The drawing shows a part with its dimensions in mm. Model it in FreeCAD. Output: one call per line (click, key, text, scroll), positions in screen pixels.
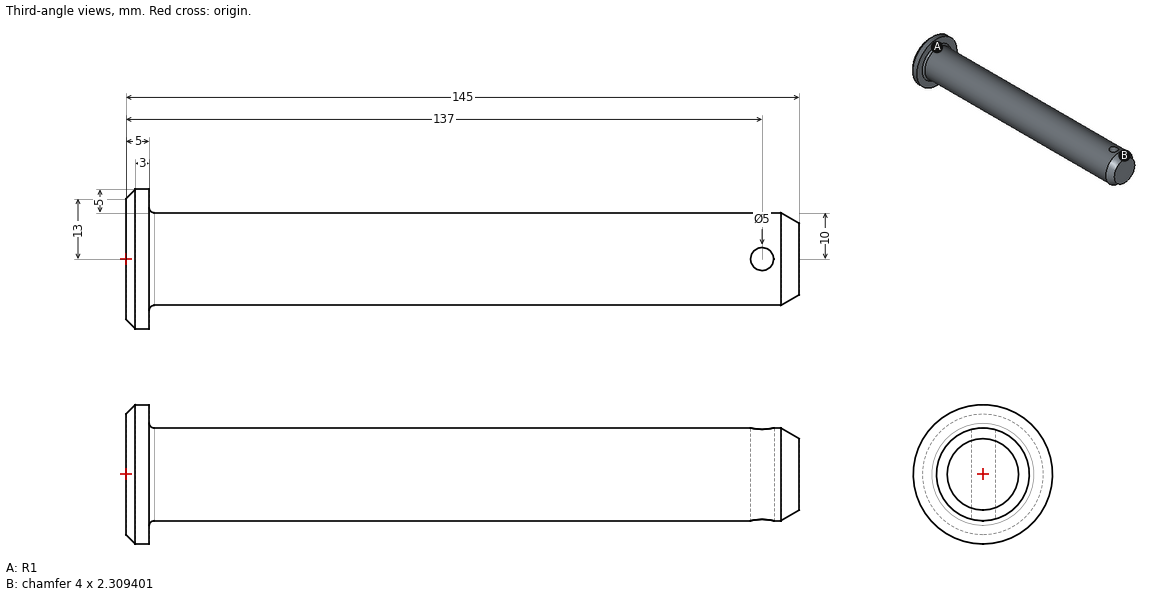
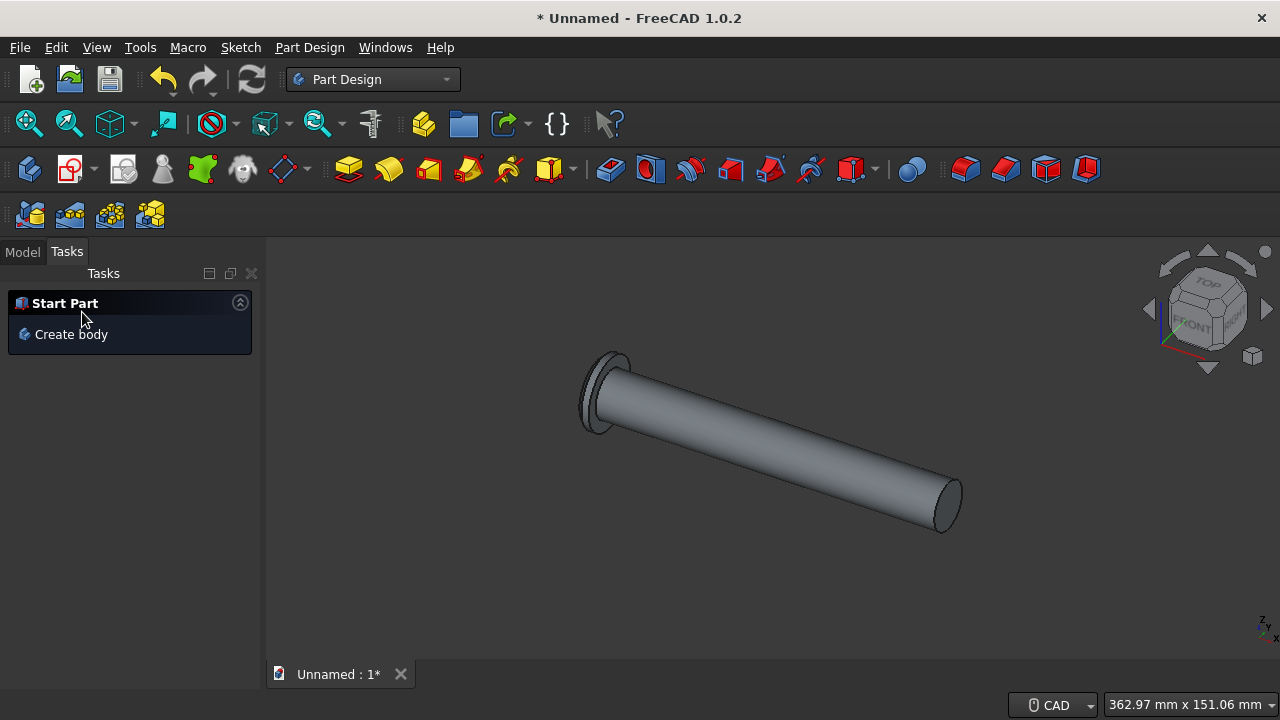
click(70, 170)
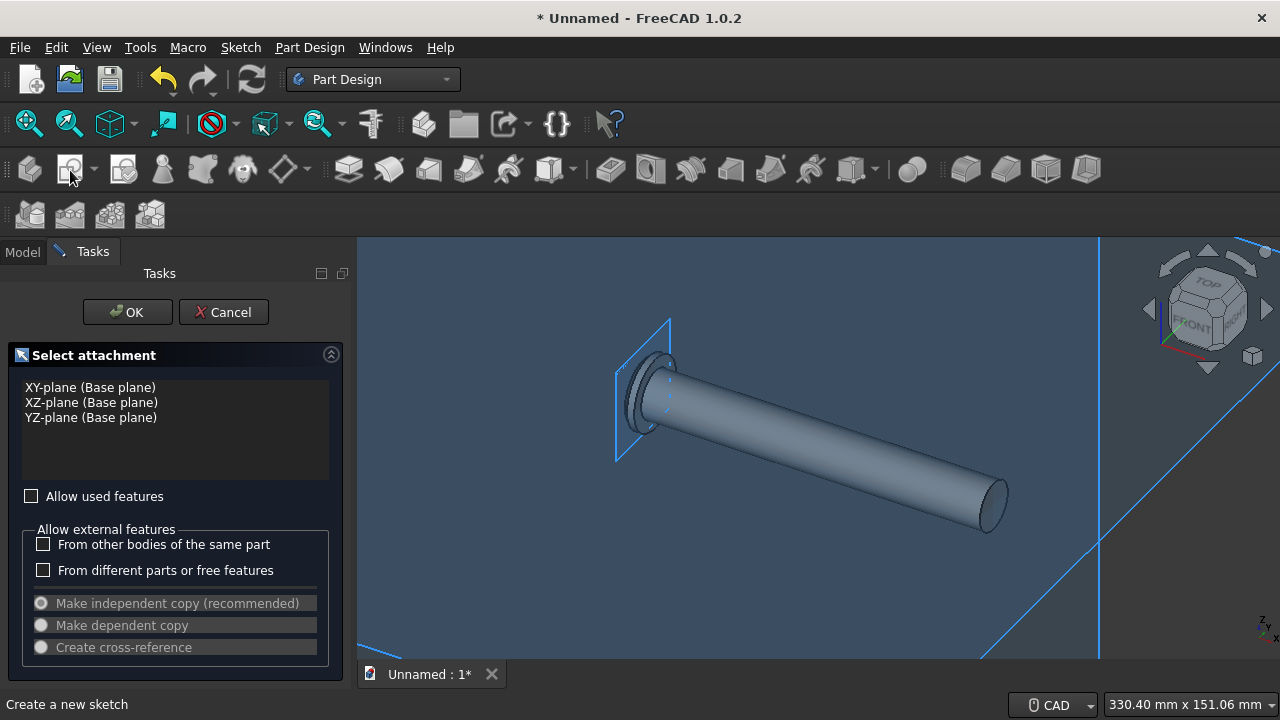
click(82, 388)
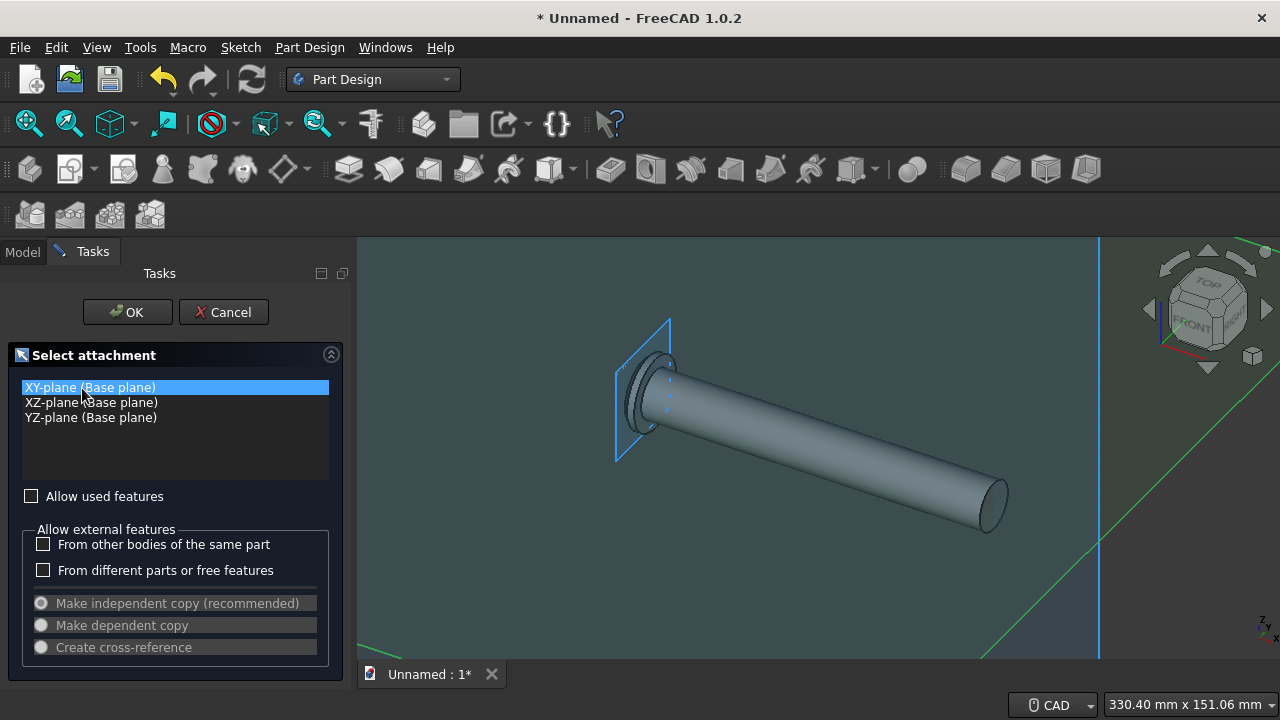
click(128, 312)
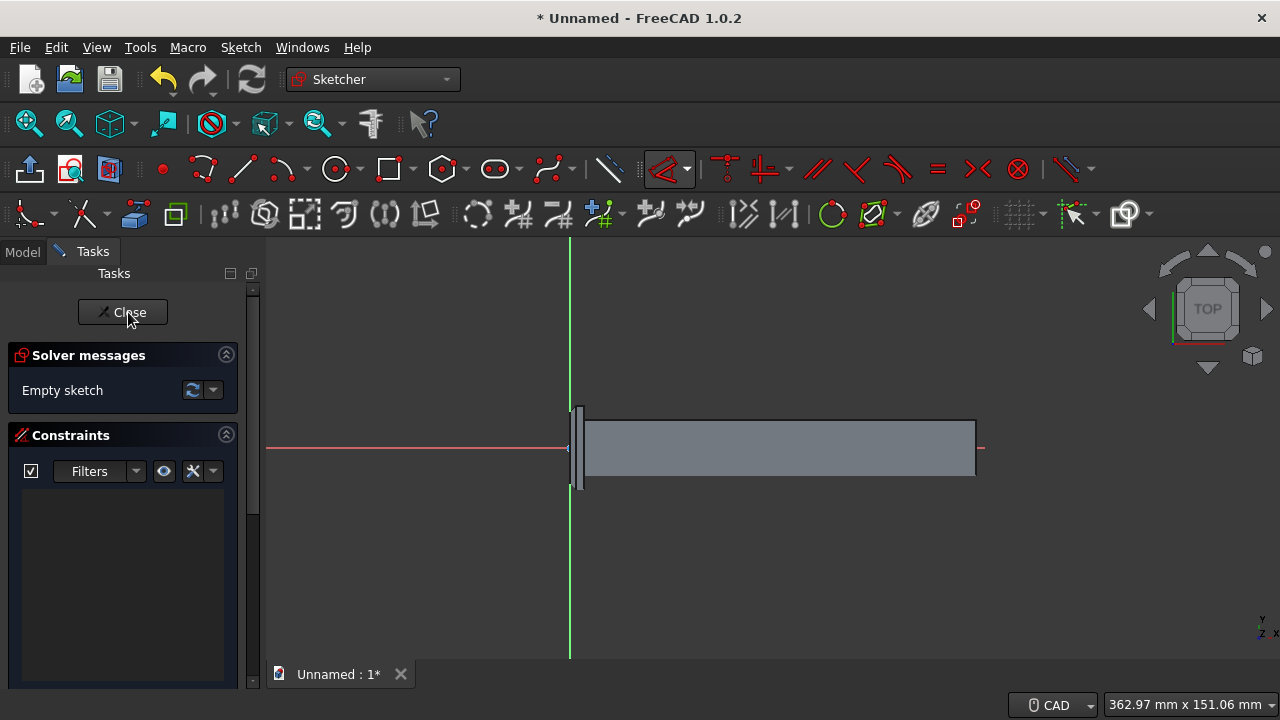
click(110, 170)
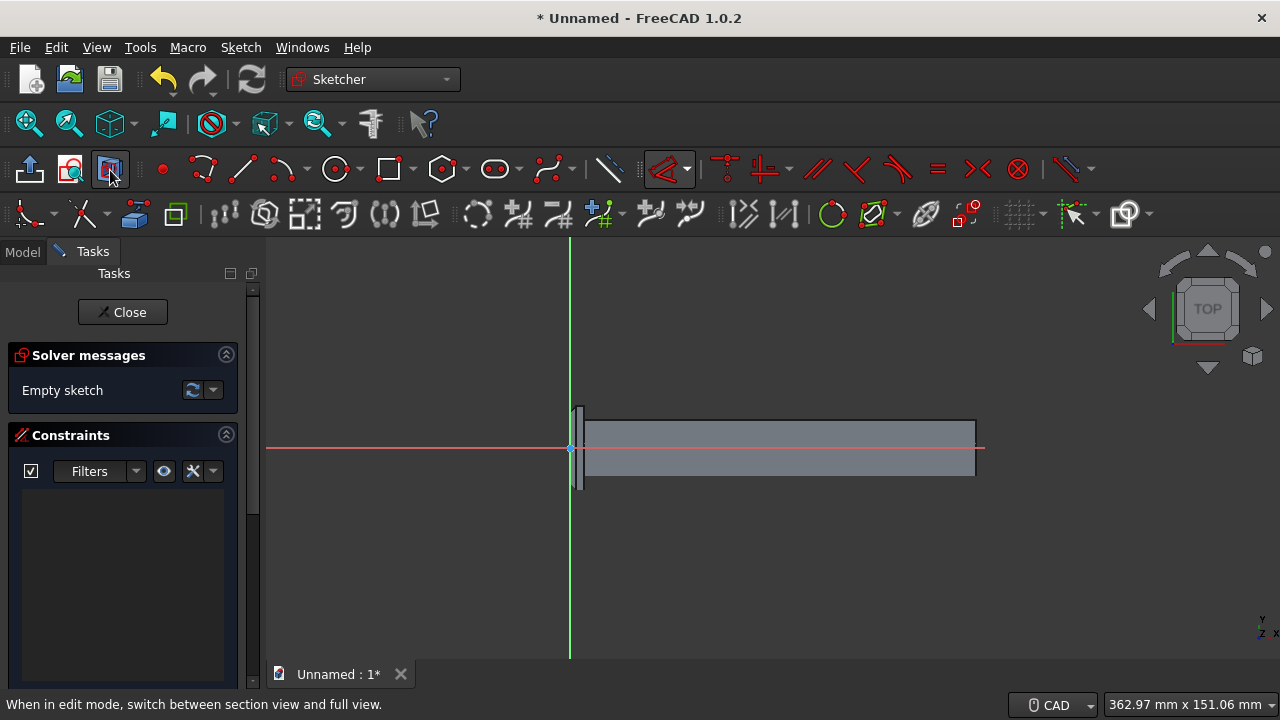
scroll(966, 448, up, 15)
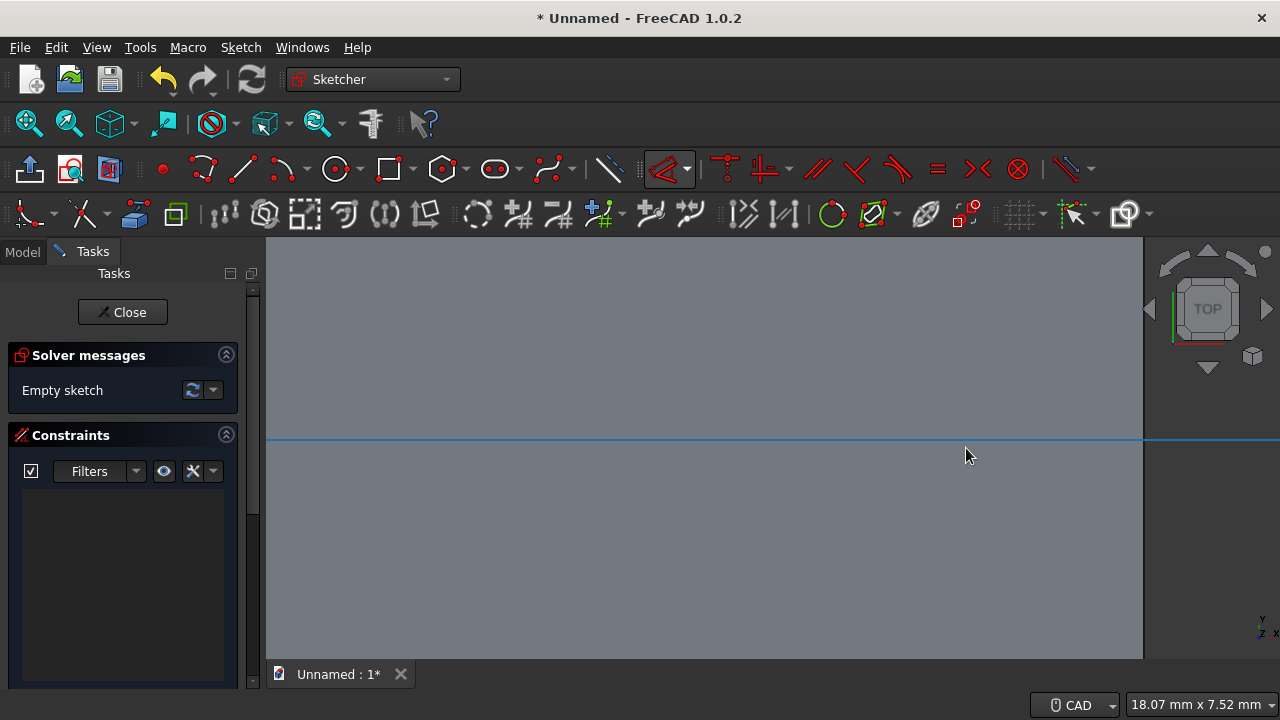
key(g)
key(c)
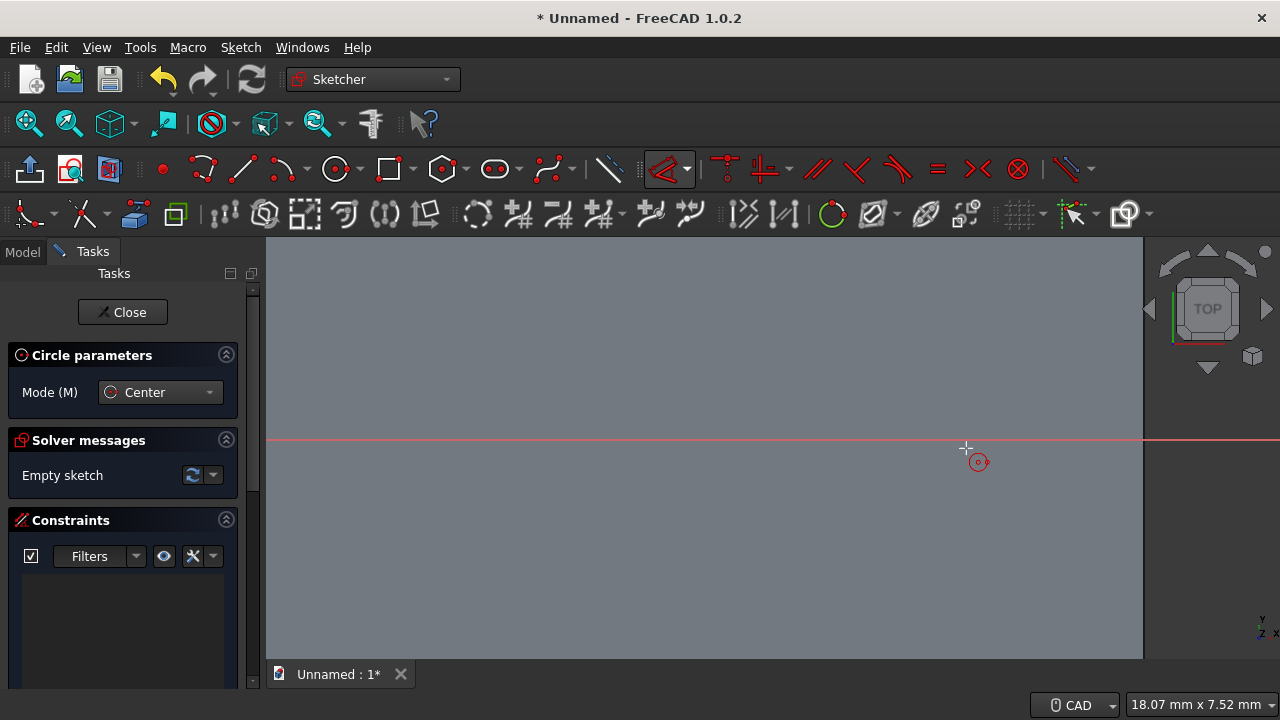
click(695, 440)
click(795, 341)
key(Escape)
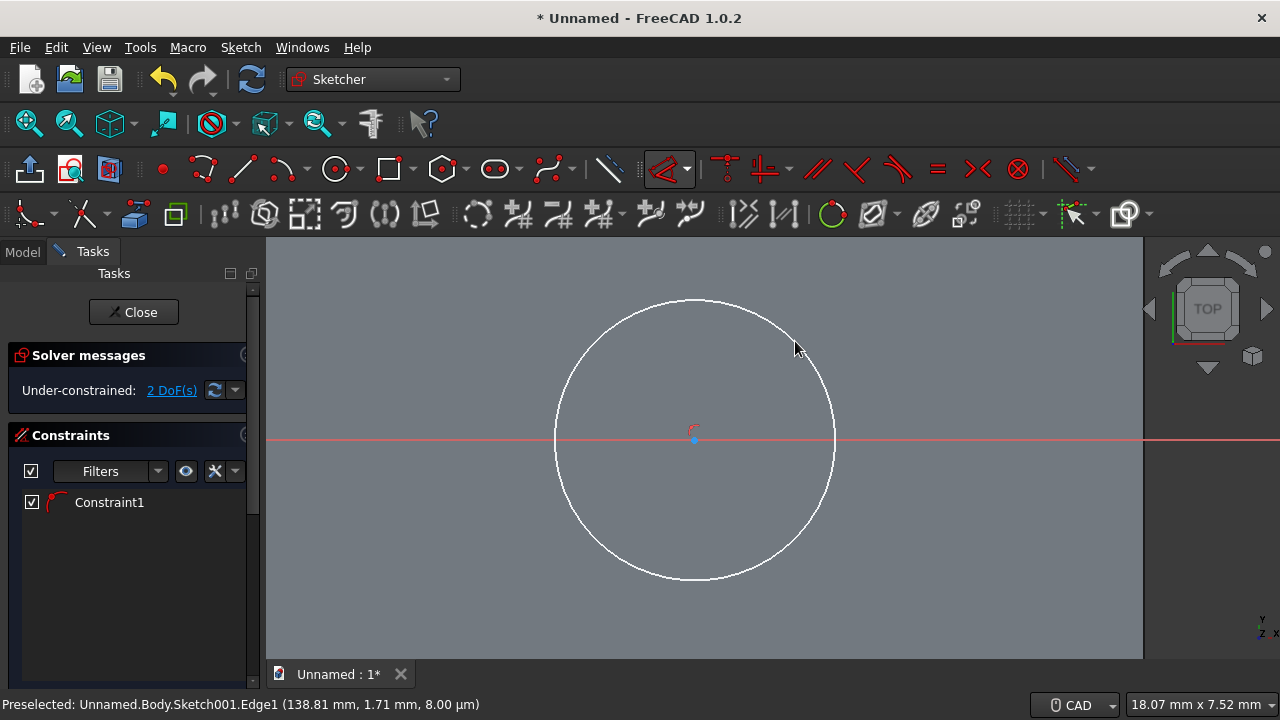
click(794, 341)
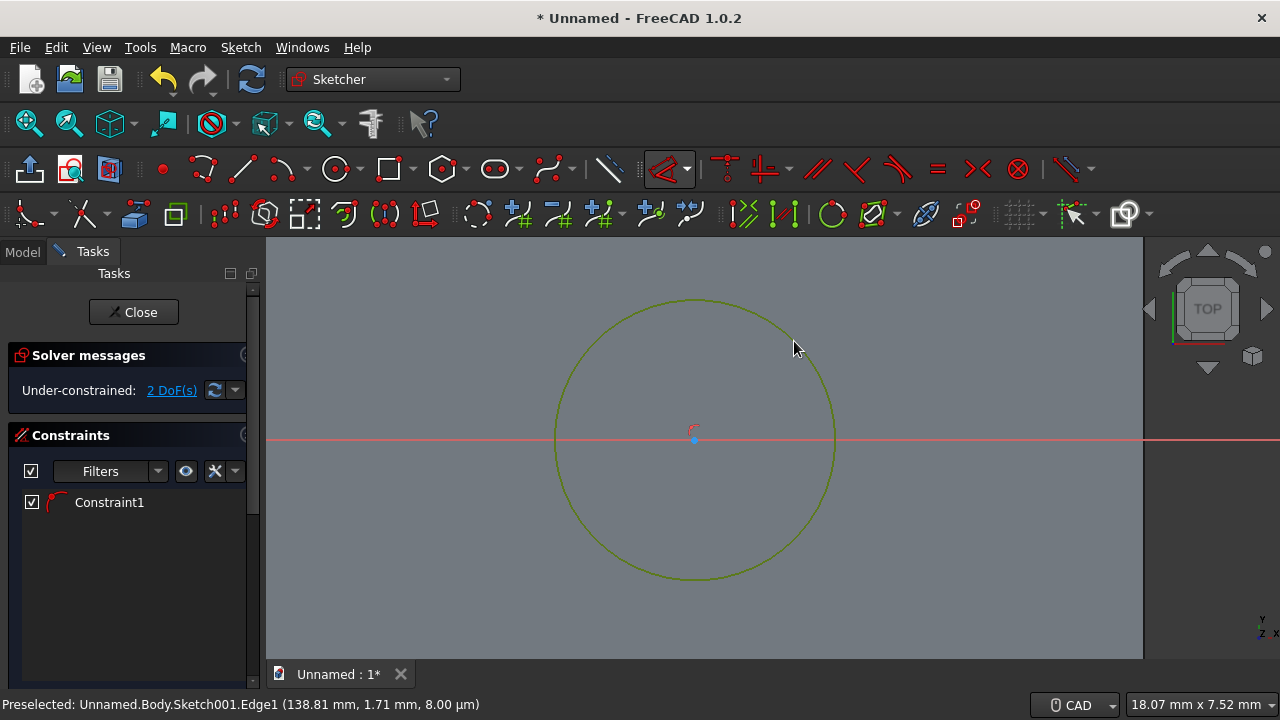
key(k)
key(o)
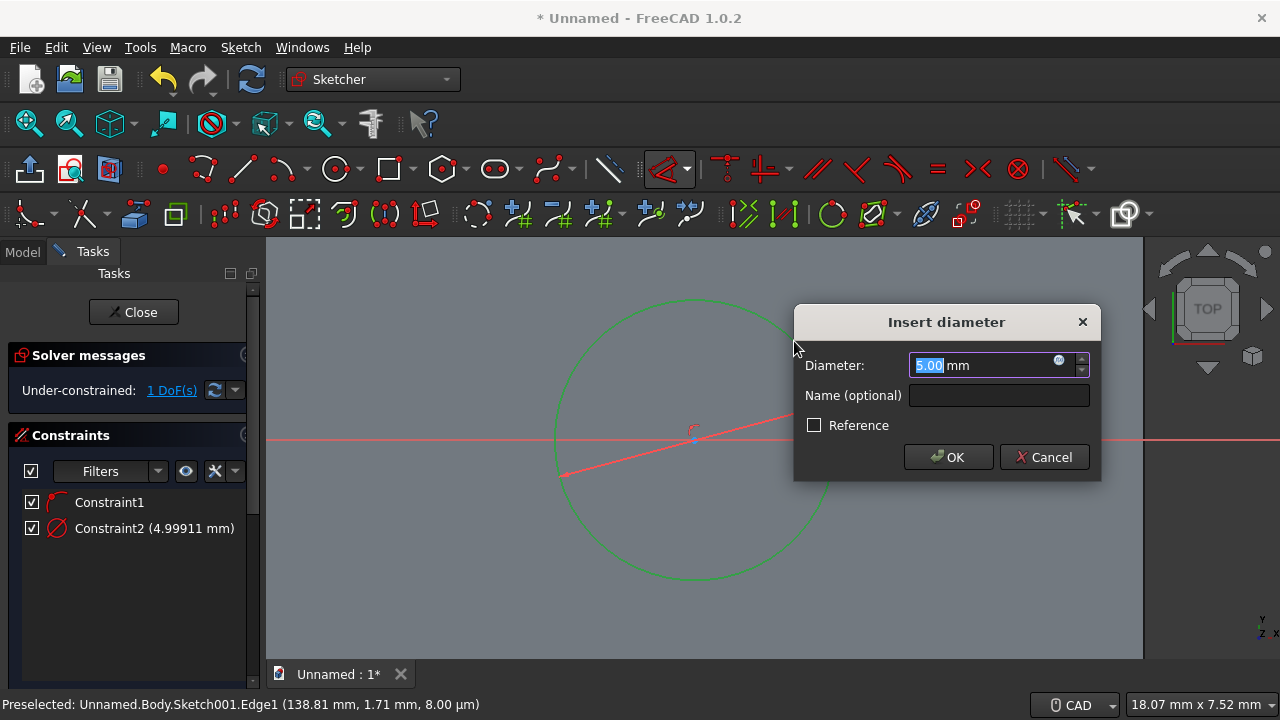
text(5)
key(Return)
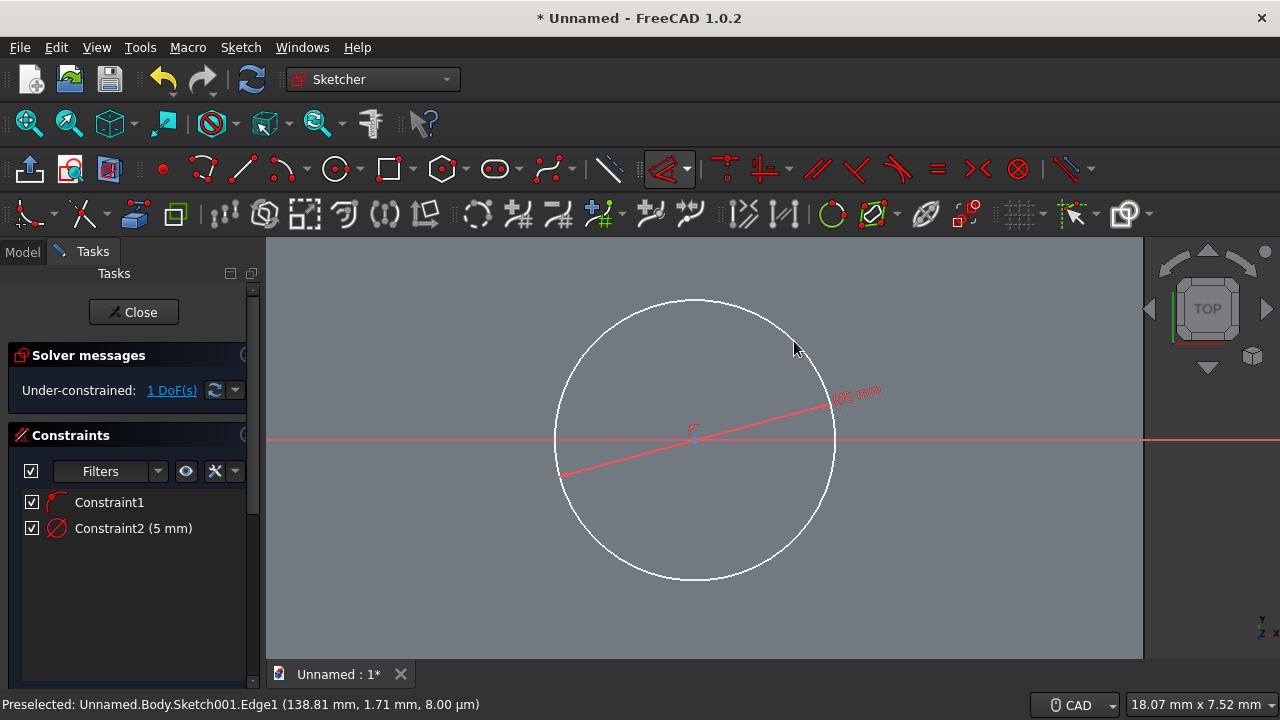
click(695, 440)